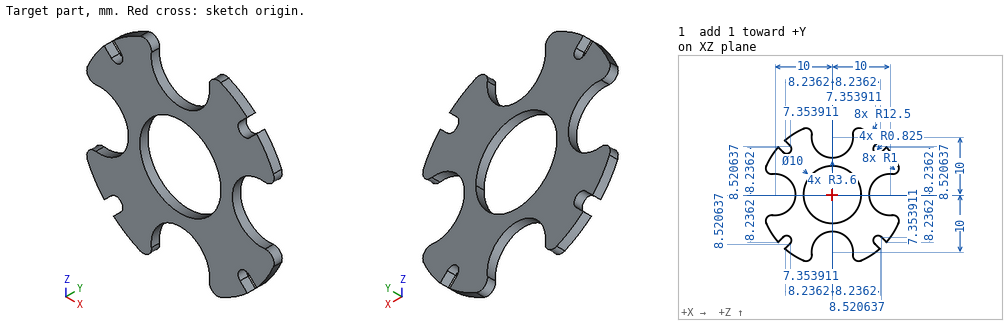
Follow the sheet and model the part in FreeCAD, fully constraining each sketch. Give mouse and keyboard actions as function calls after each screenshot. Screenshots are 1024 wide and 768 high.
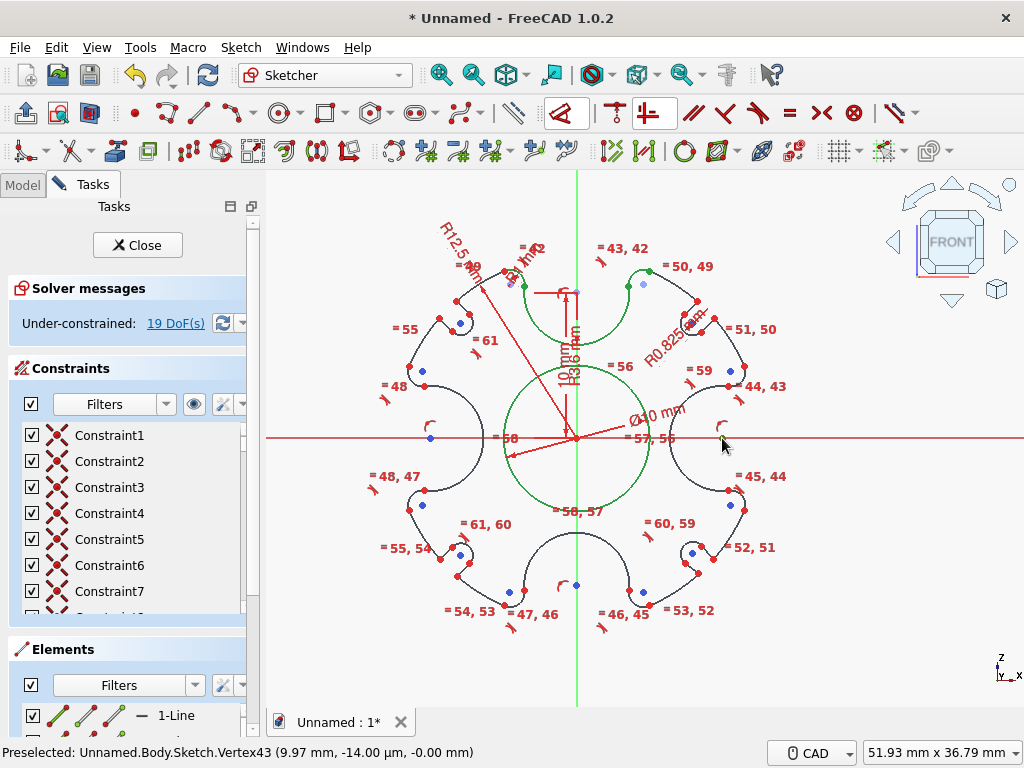
key(l)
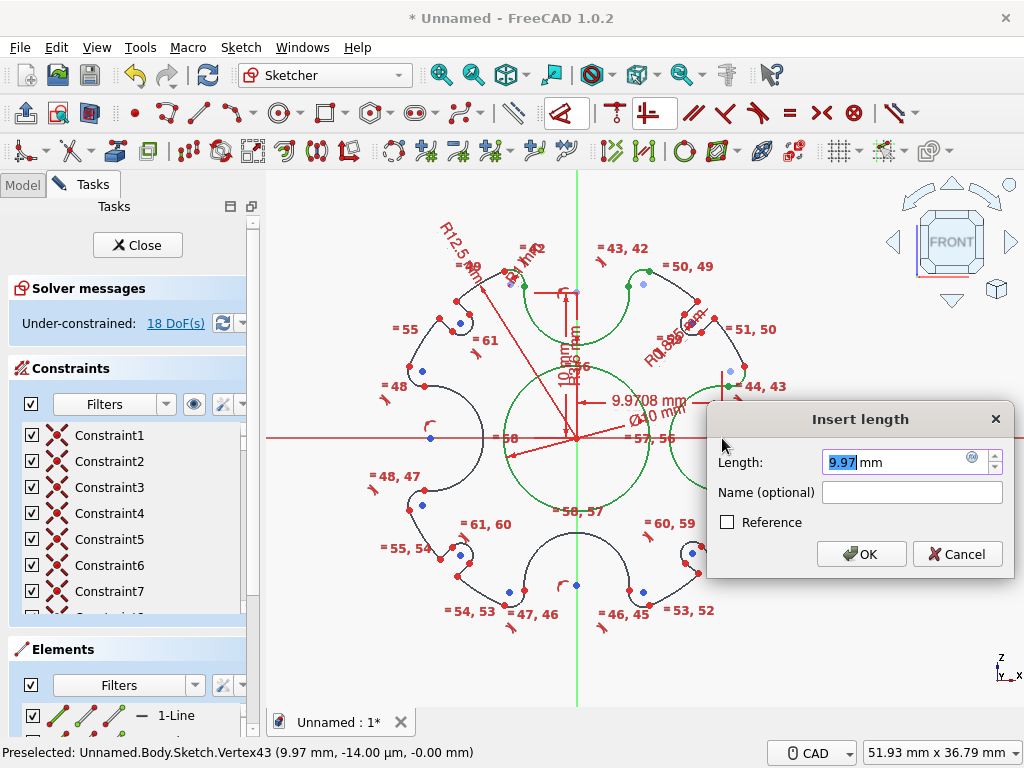
text(10)
key(Return)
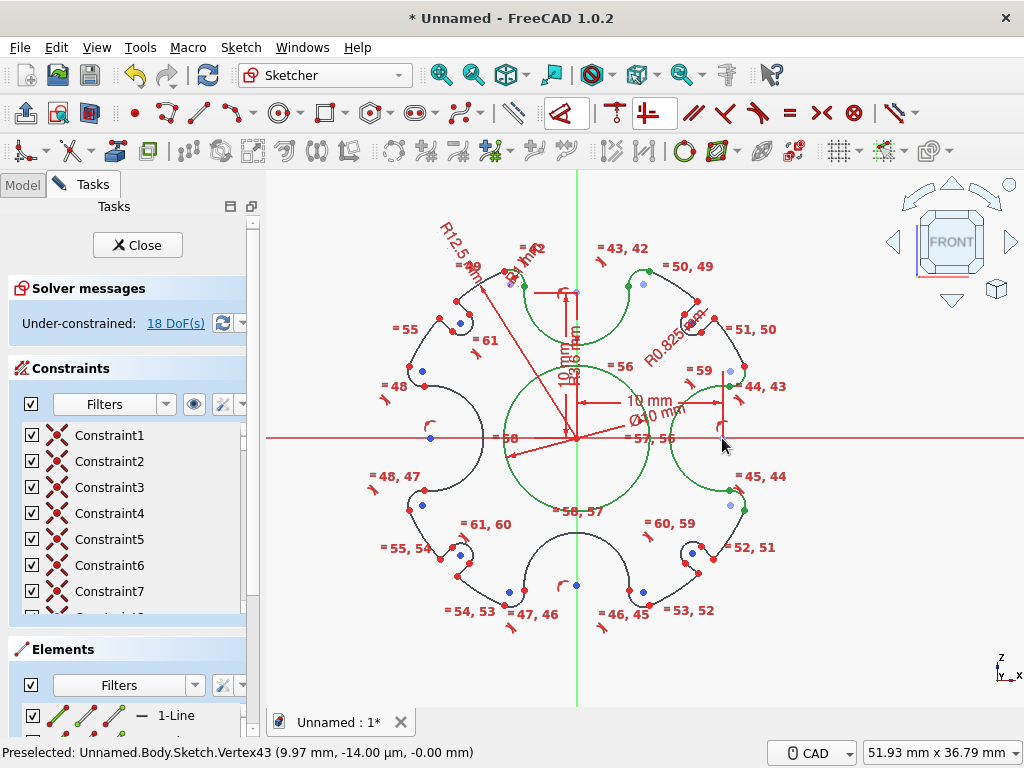
click(577, 585)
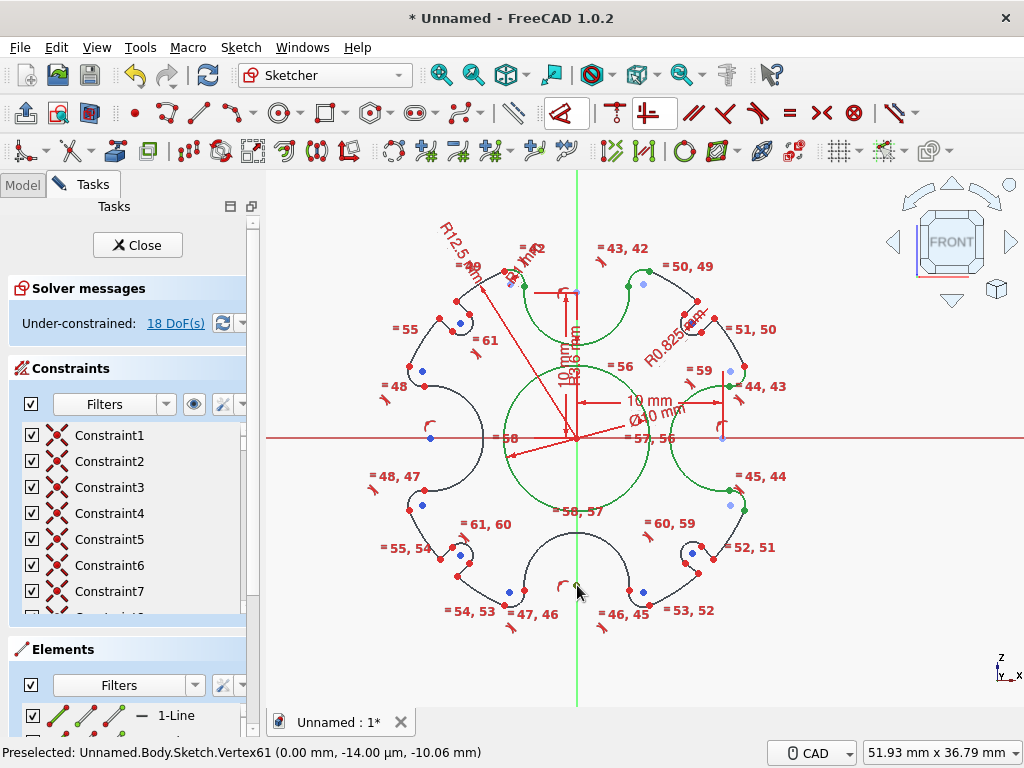
click(584, 114)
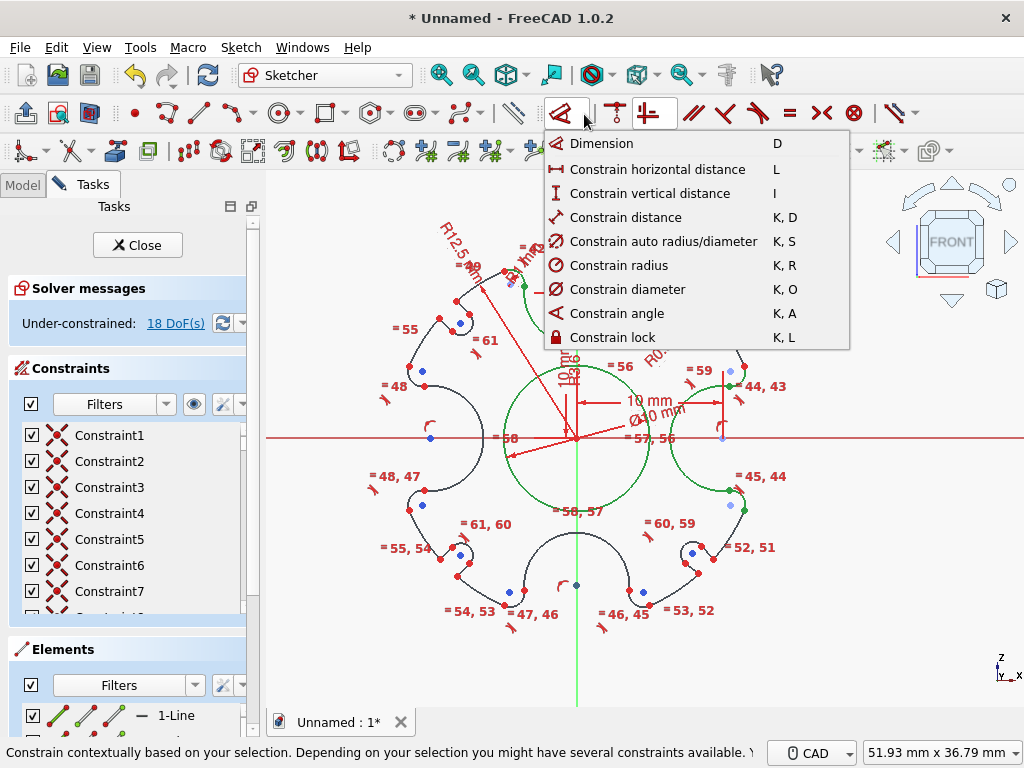
click(697, 193)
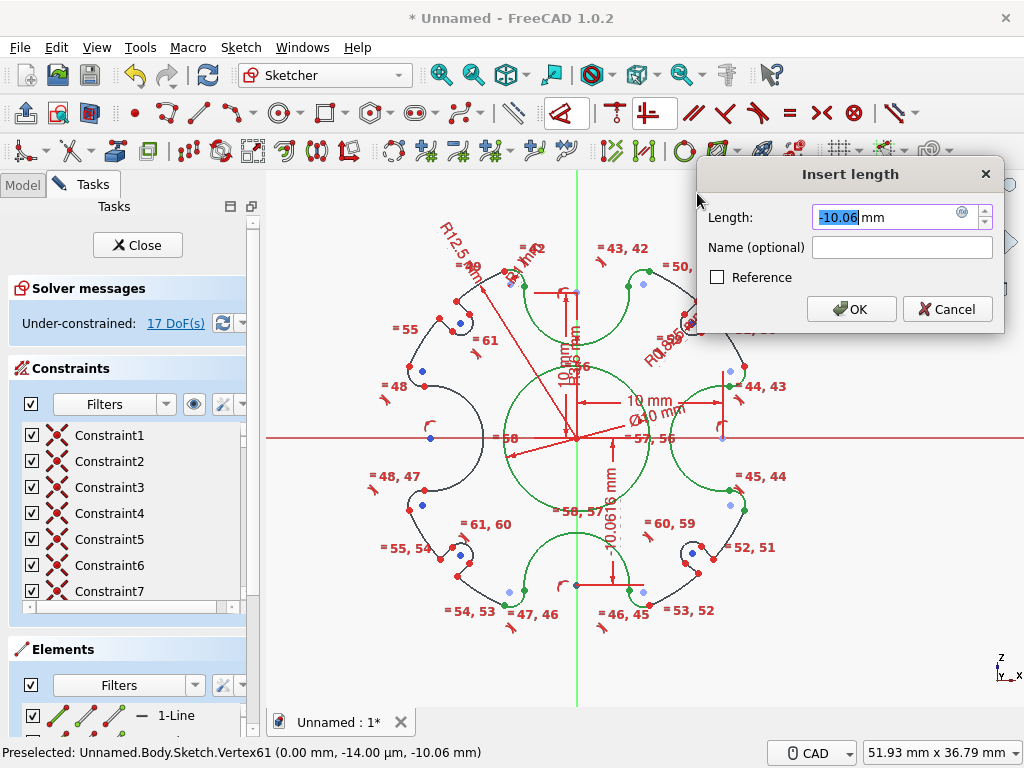
text(-10)
key(Return)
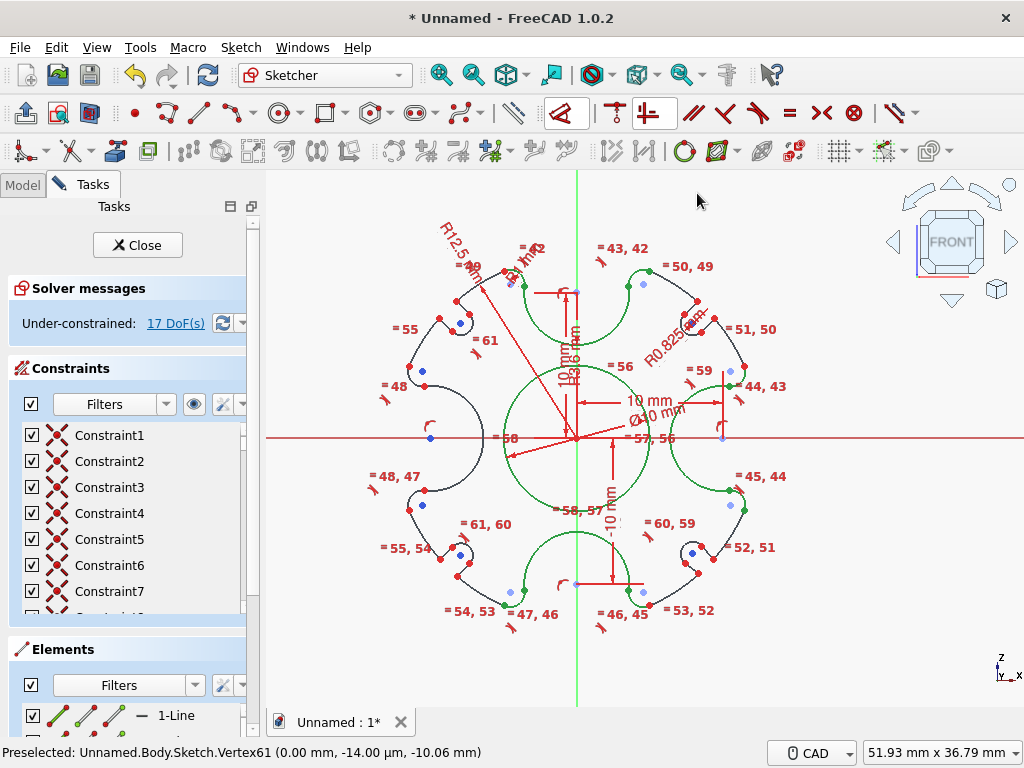
click(431, 438)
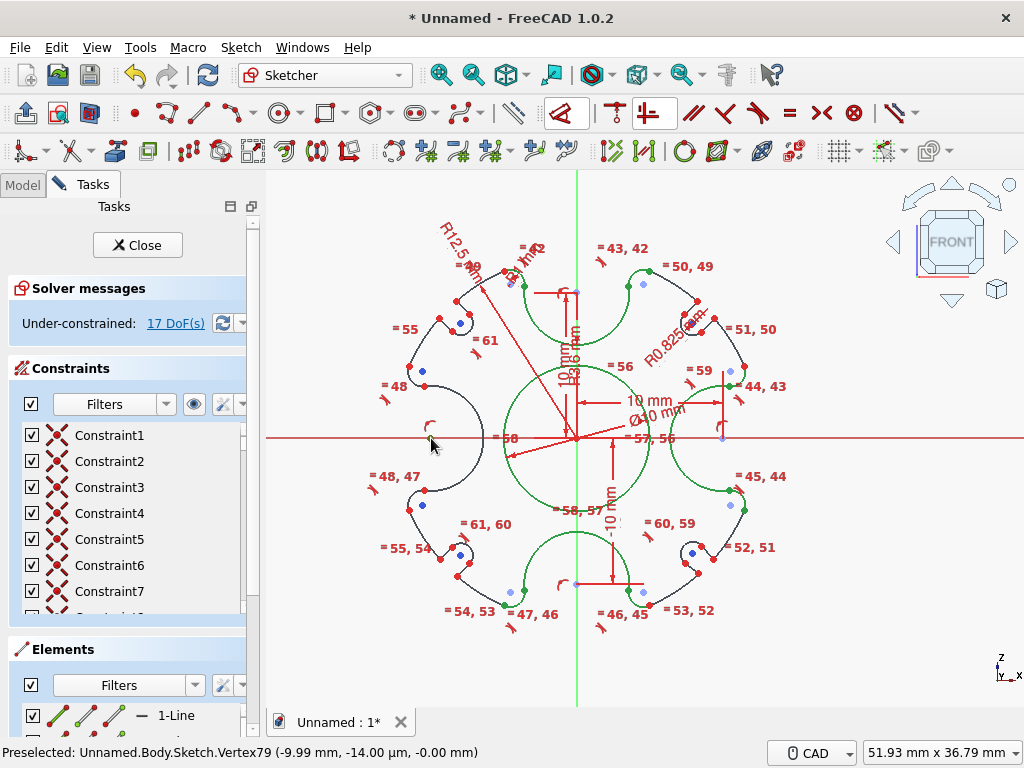
click(584, 114)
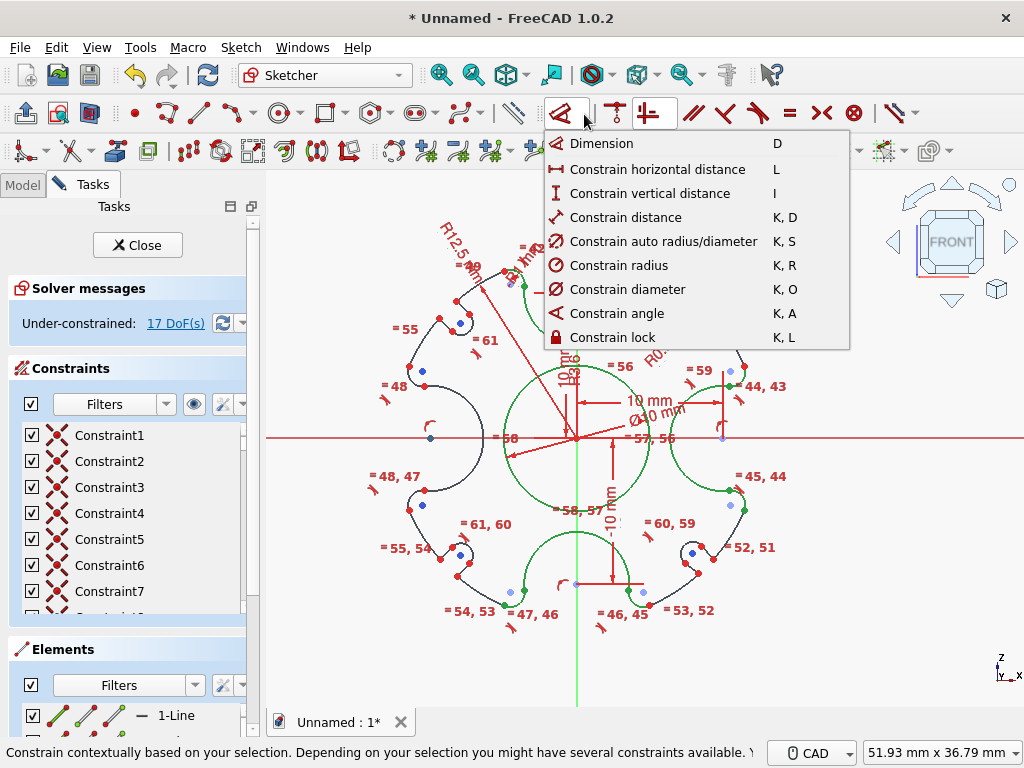
click(697, 169)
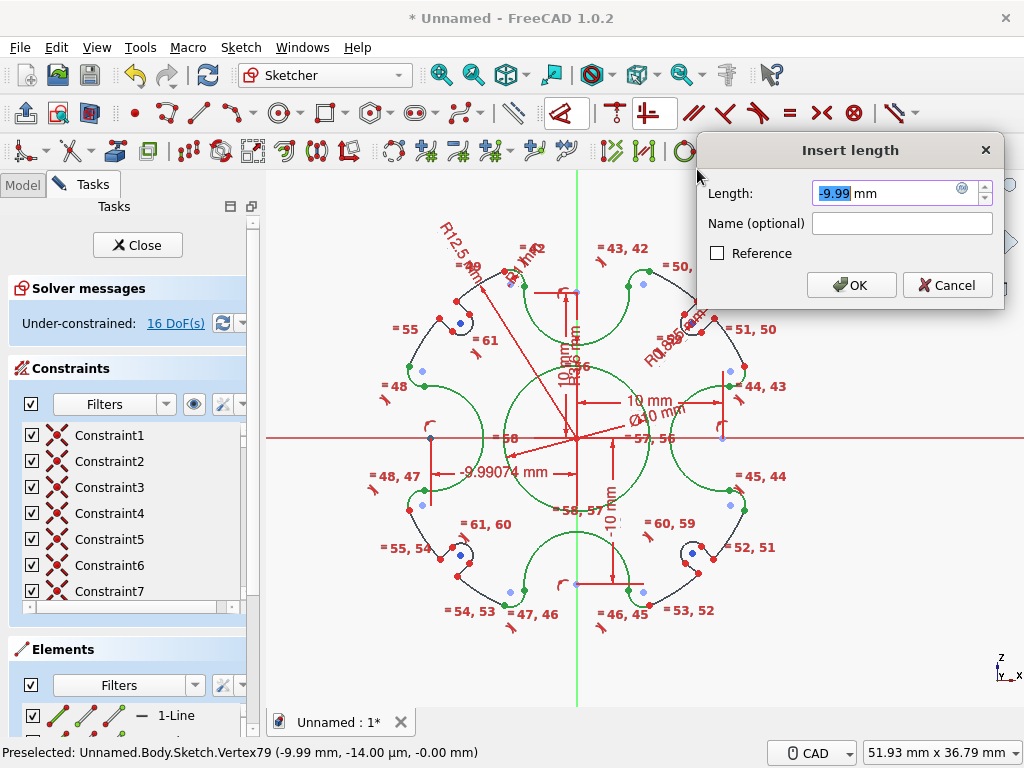
text(-10)
key(Return)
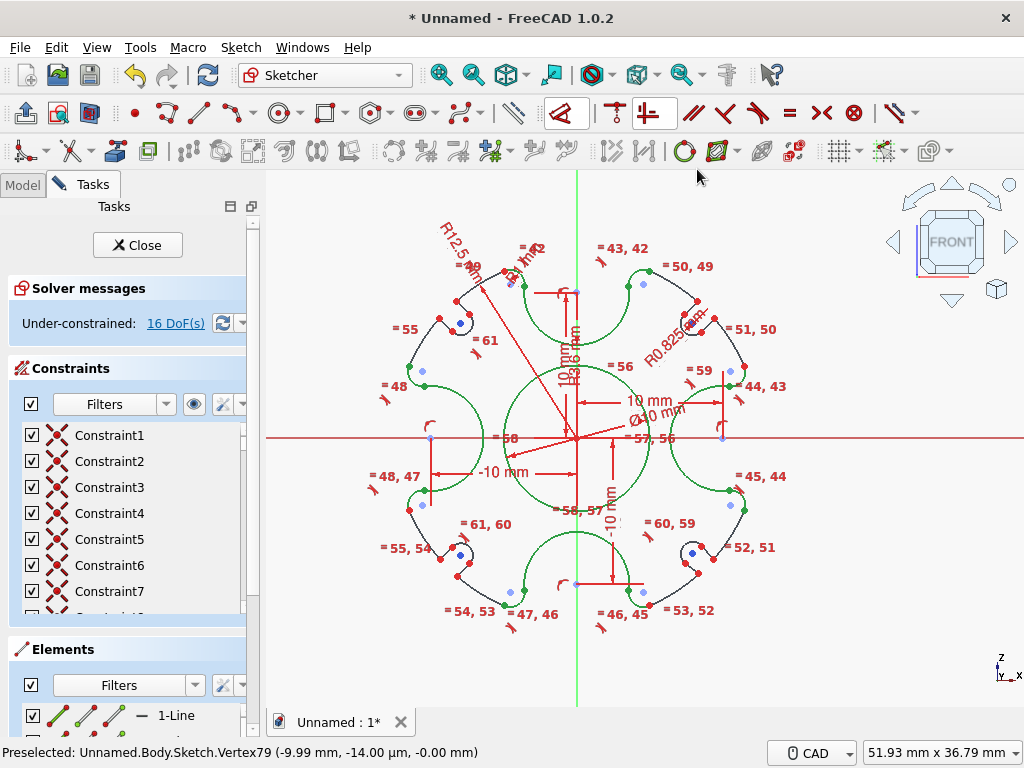
click(457, 301)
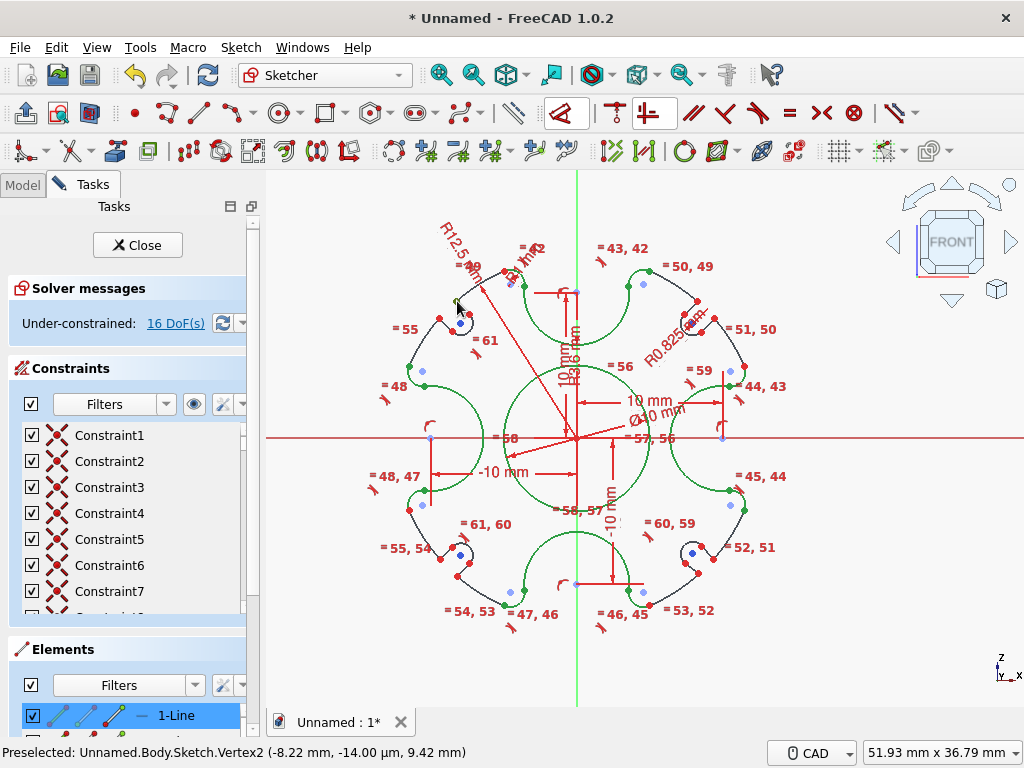
click(584, 114)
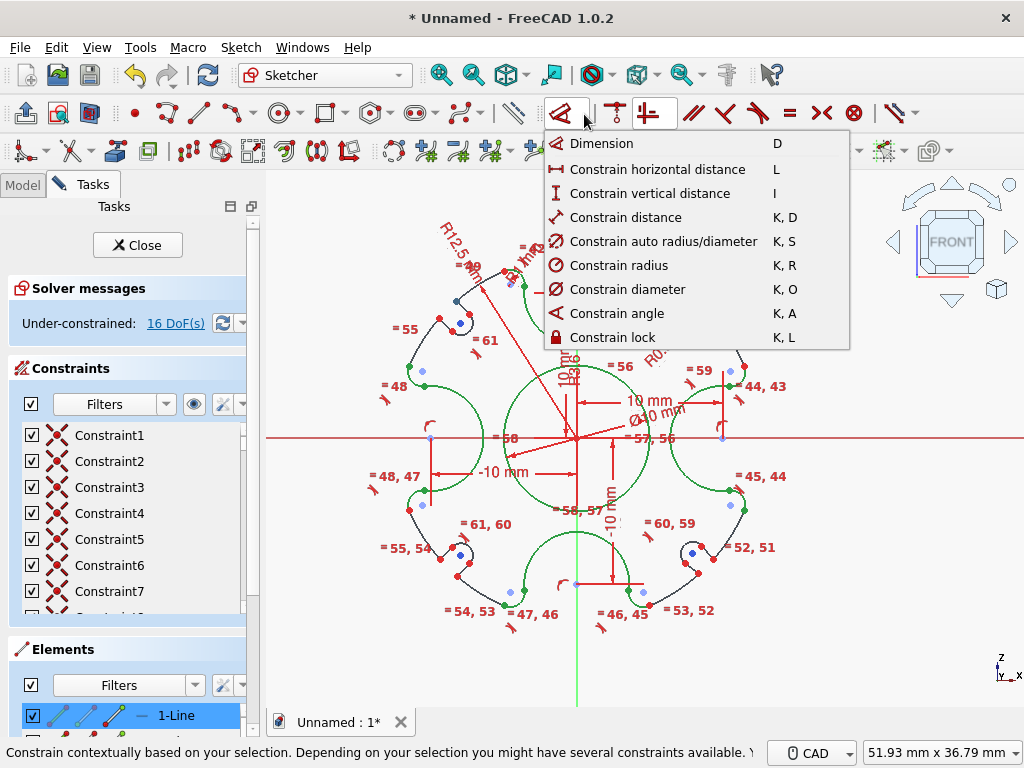
click(697, 169)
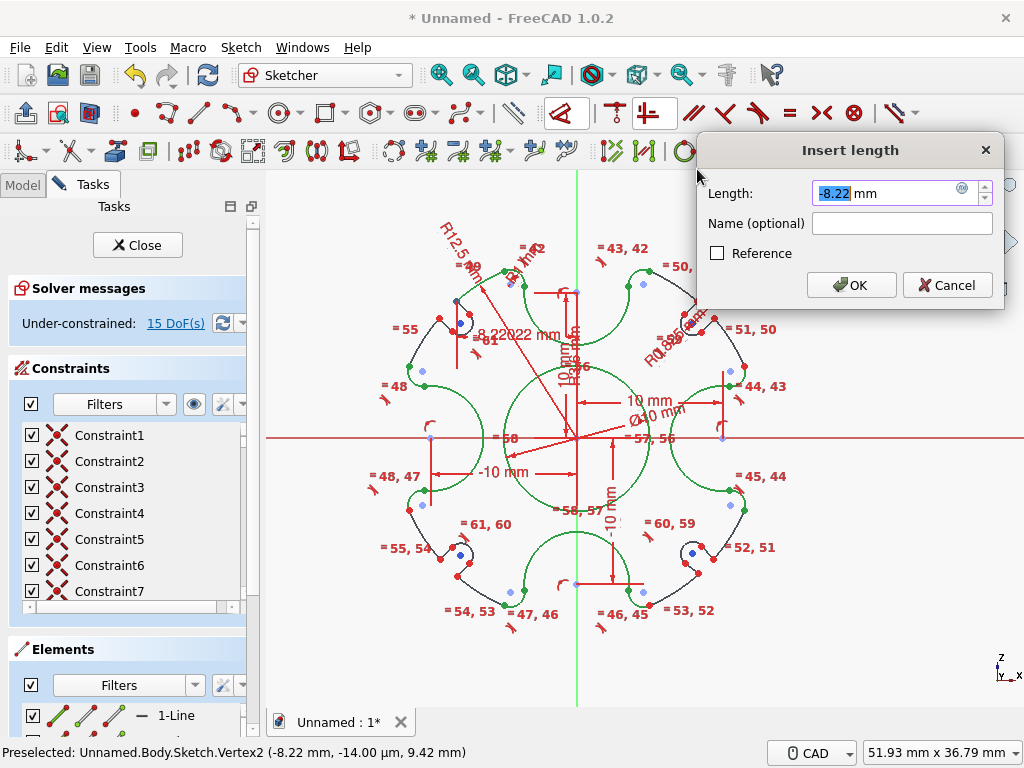
text(-8.2362)
key(Return)